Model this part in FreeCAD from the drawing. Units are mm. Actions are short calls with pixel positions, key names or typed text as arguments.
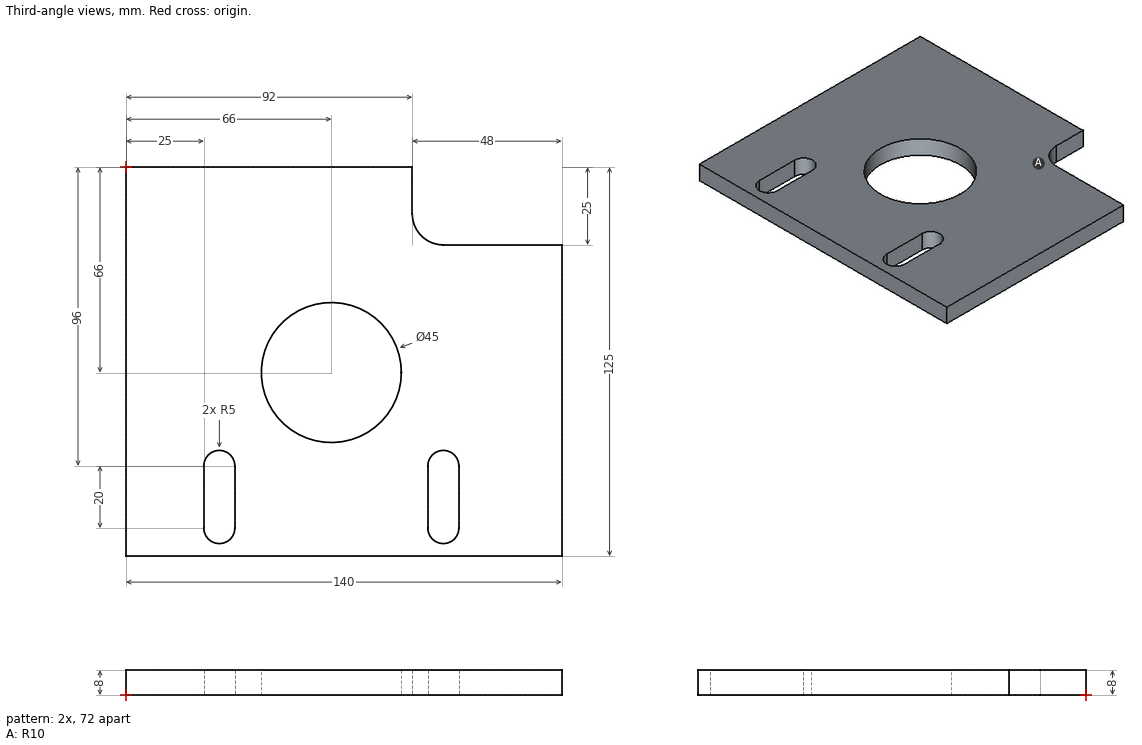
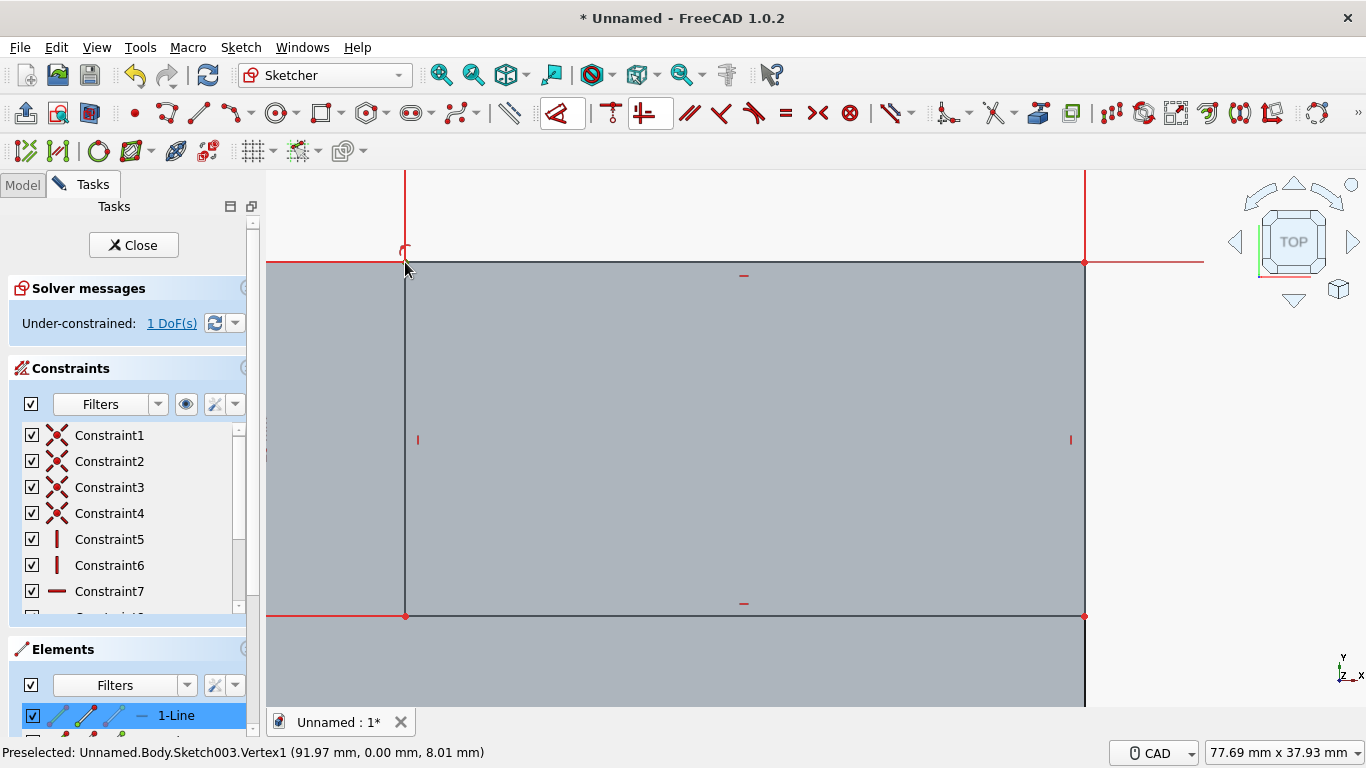
key(l)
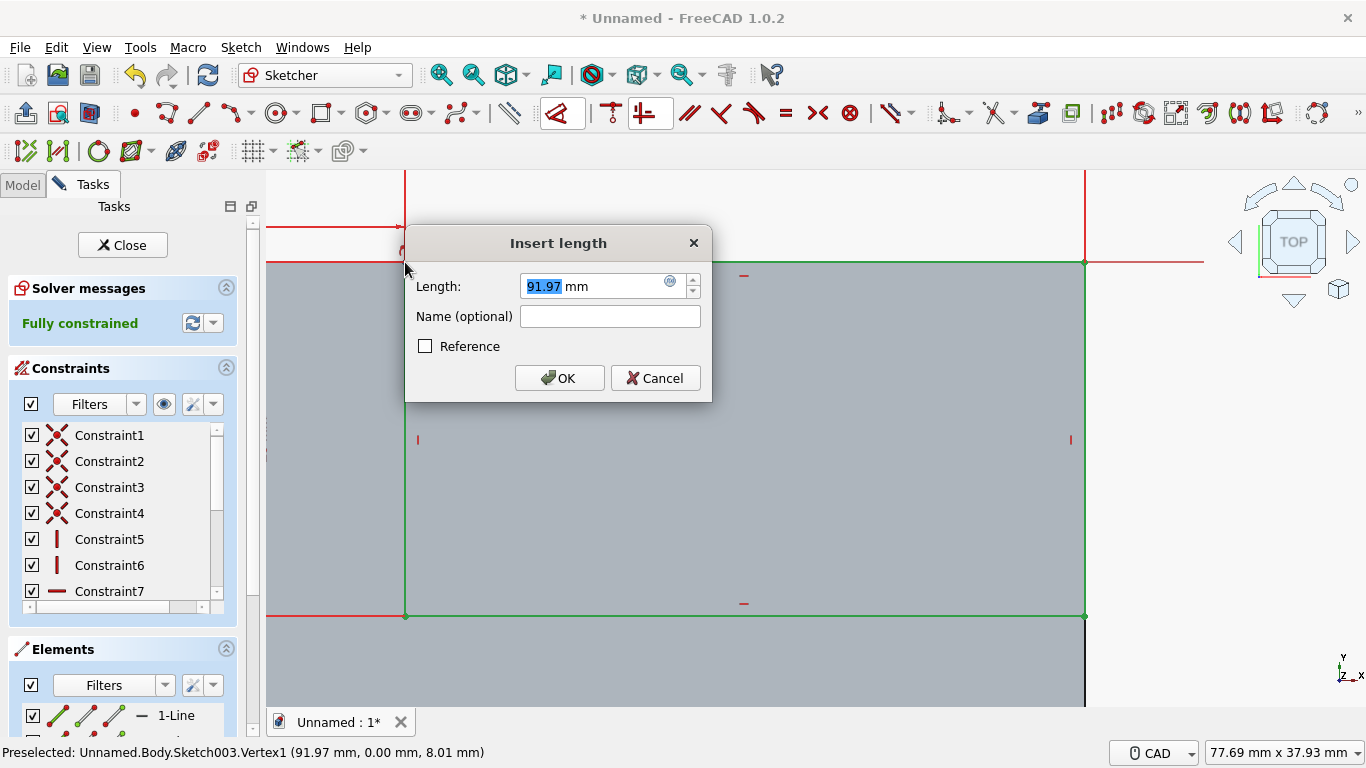
text(92)
key(Return)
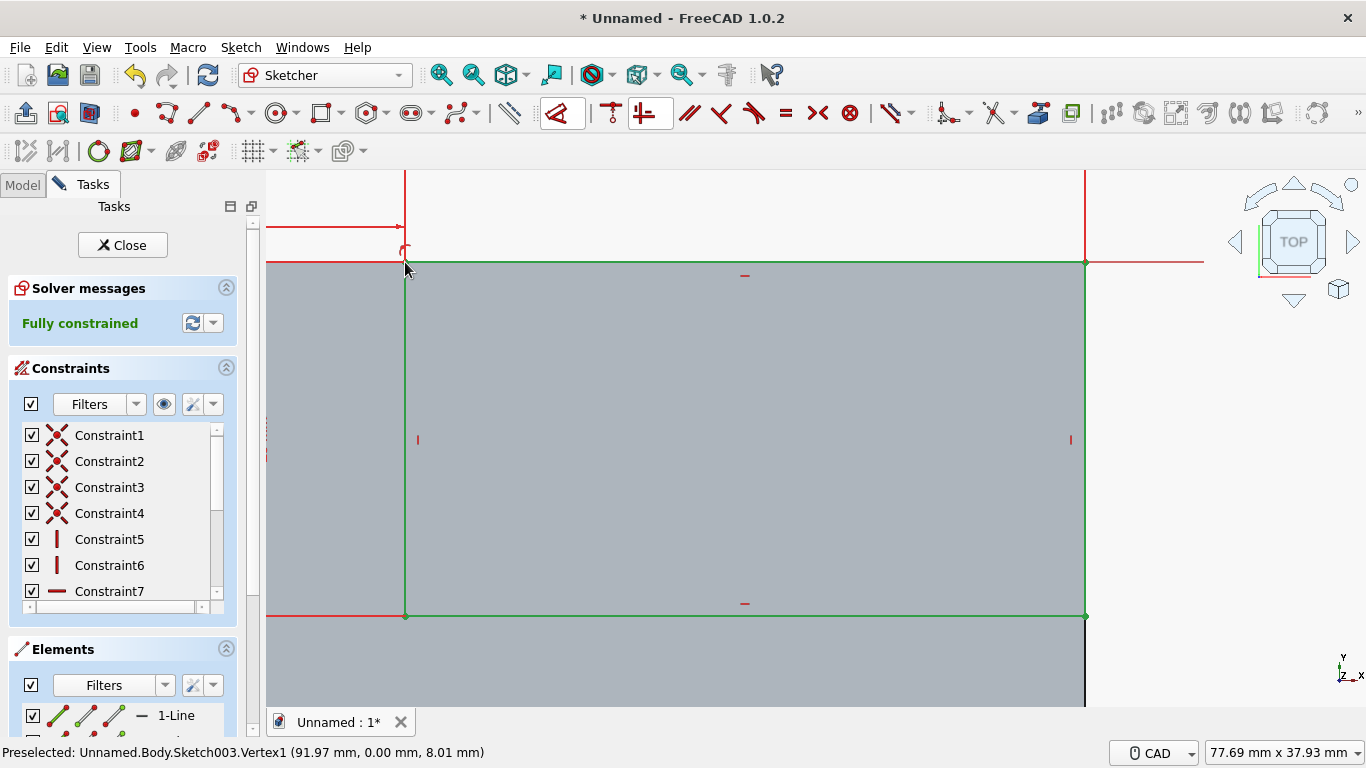
click(123, 245)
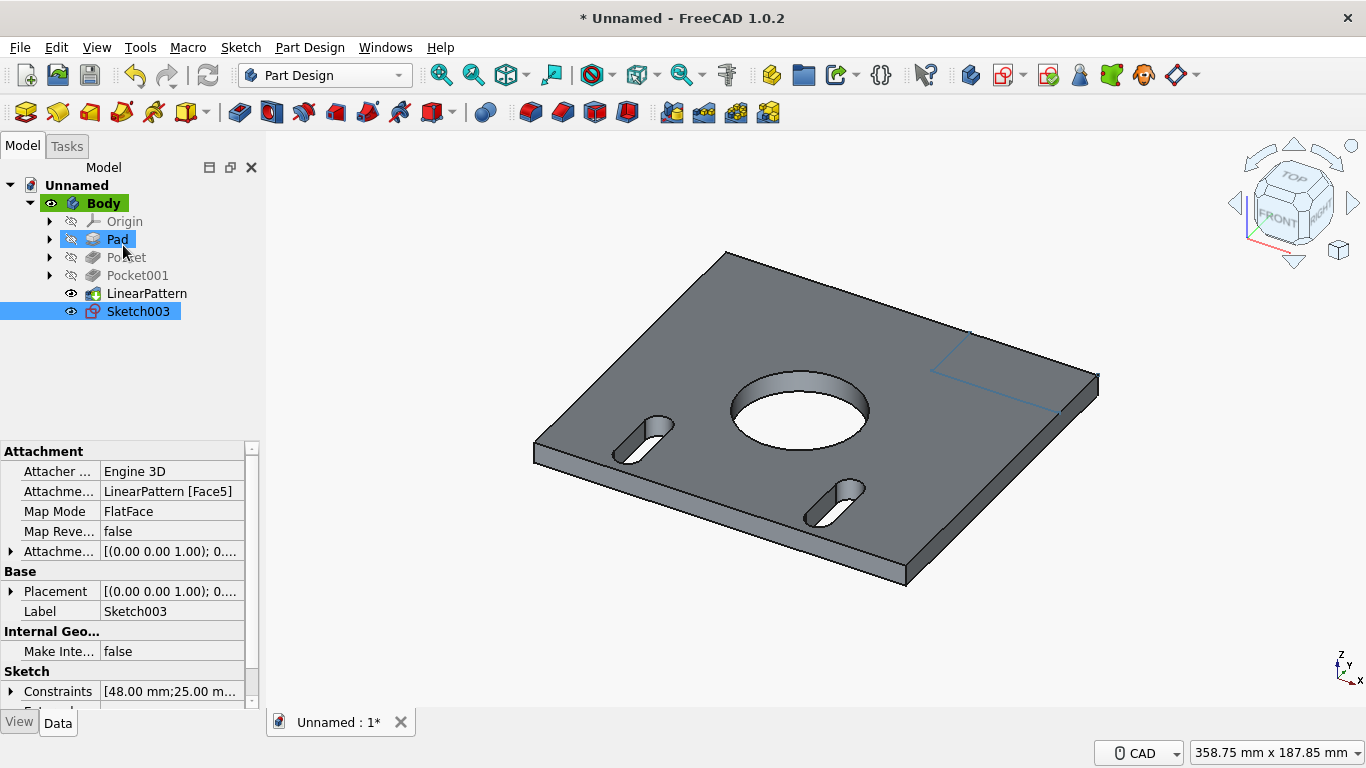
click(240, 112)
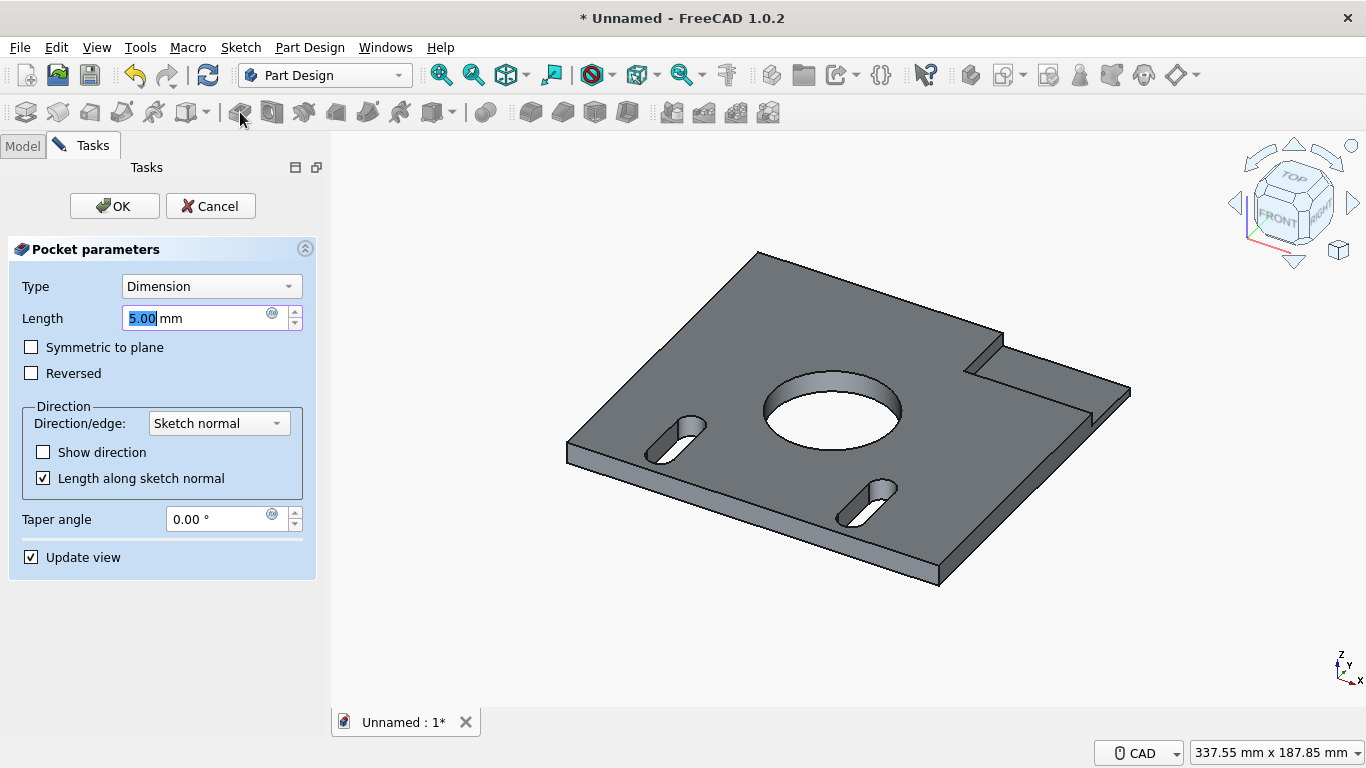
text(8)
key(Tab)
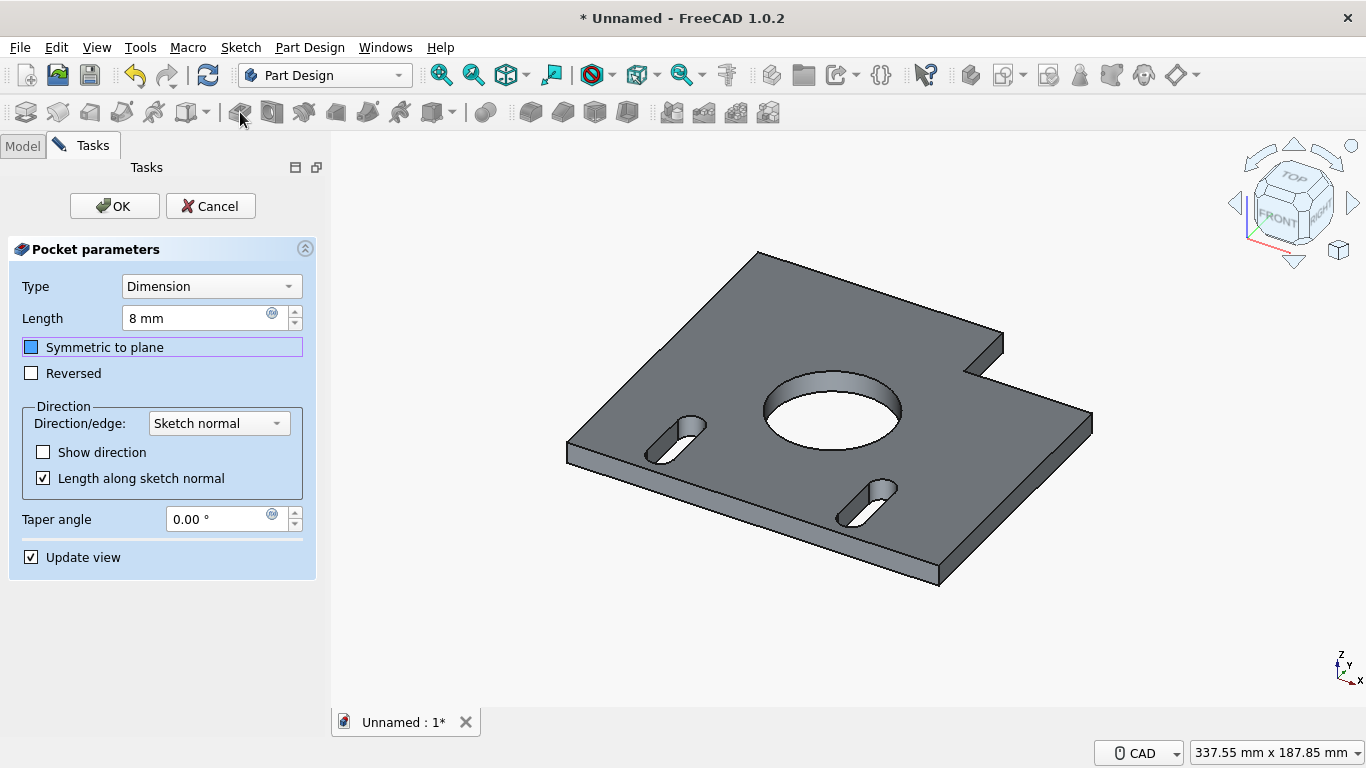
click(115, 206)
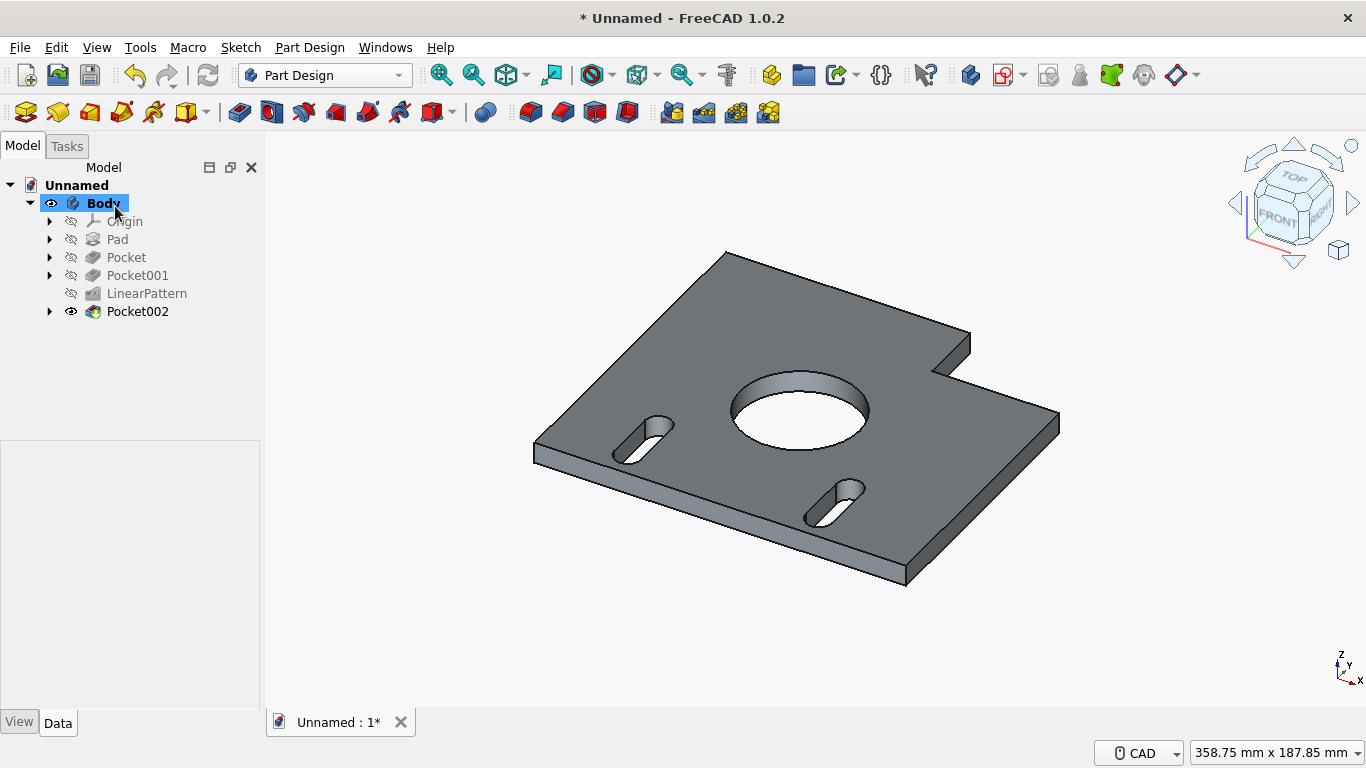
key(0)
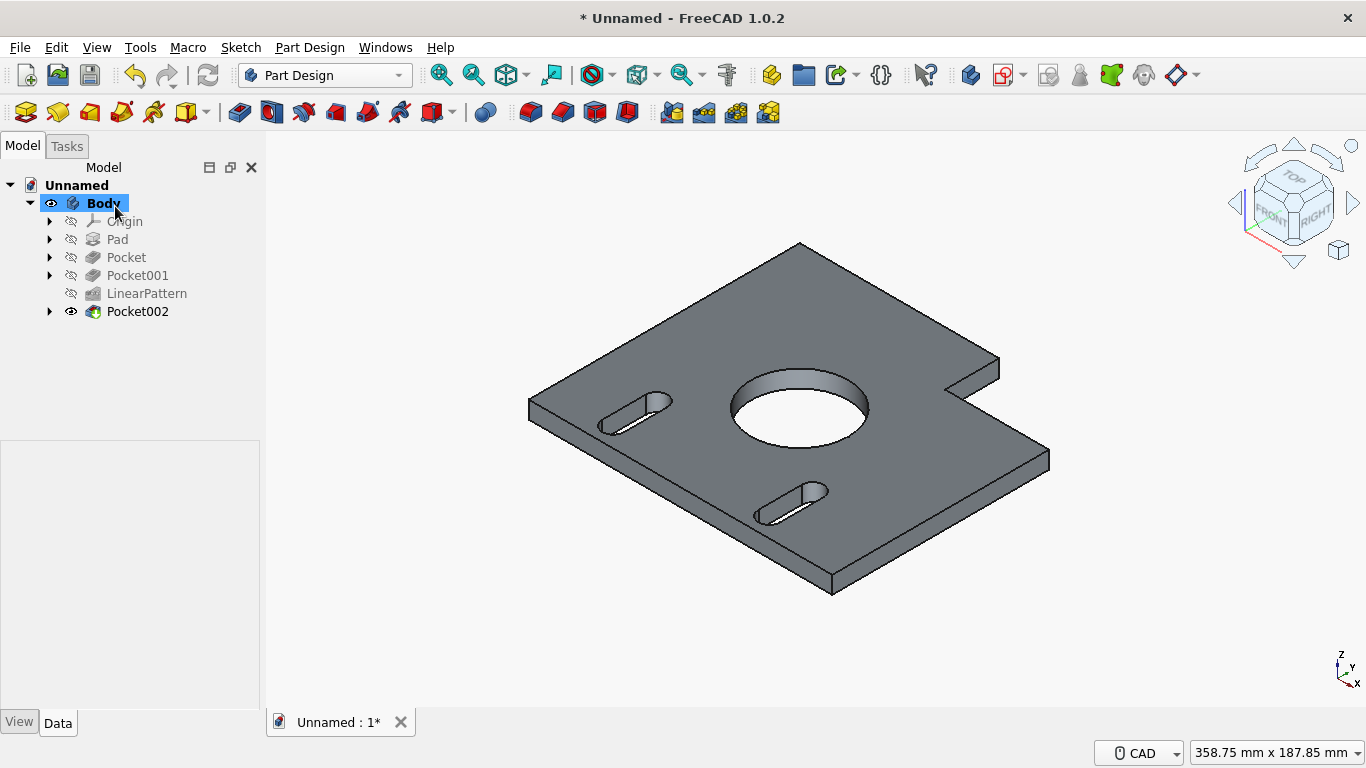
key(2)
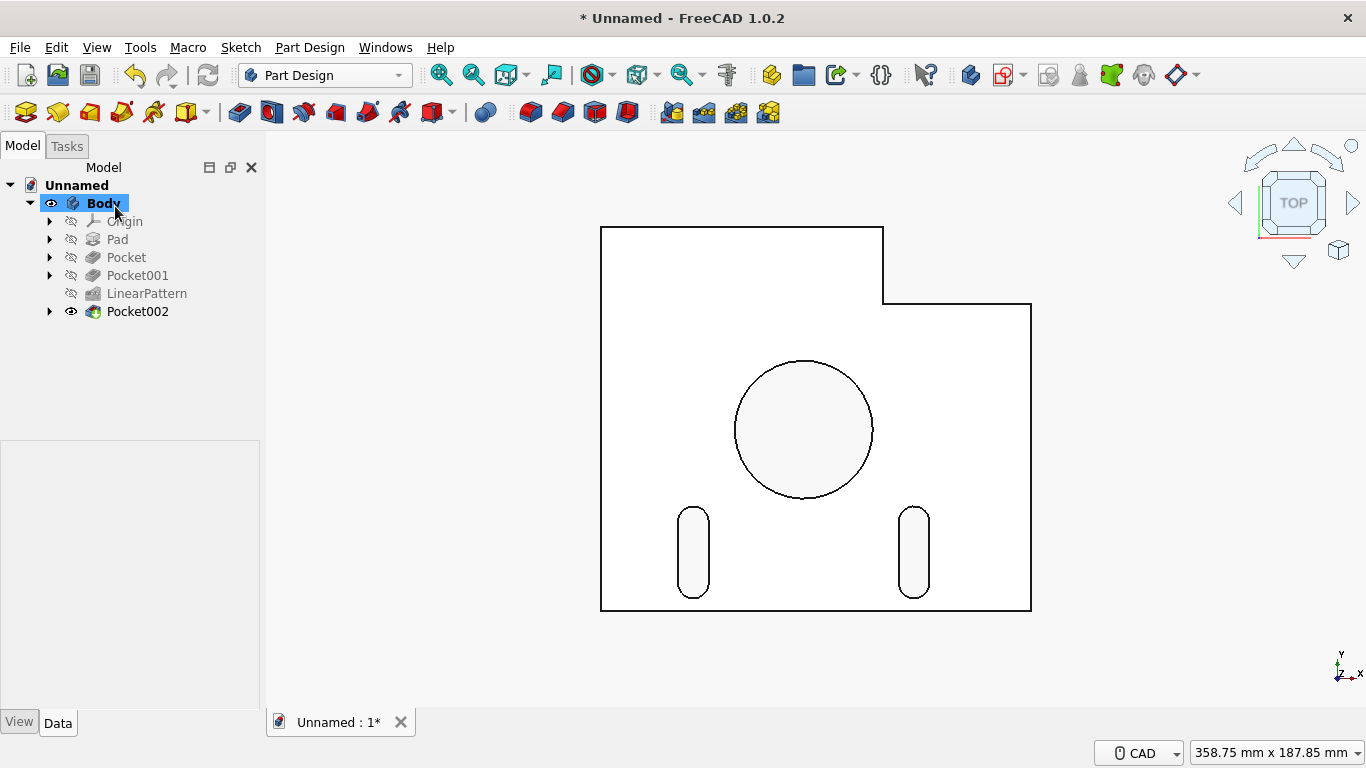
key(1)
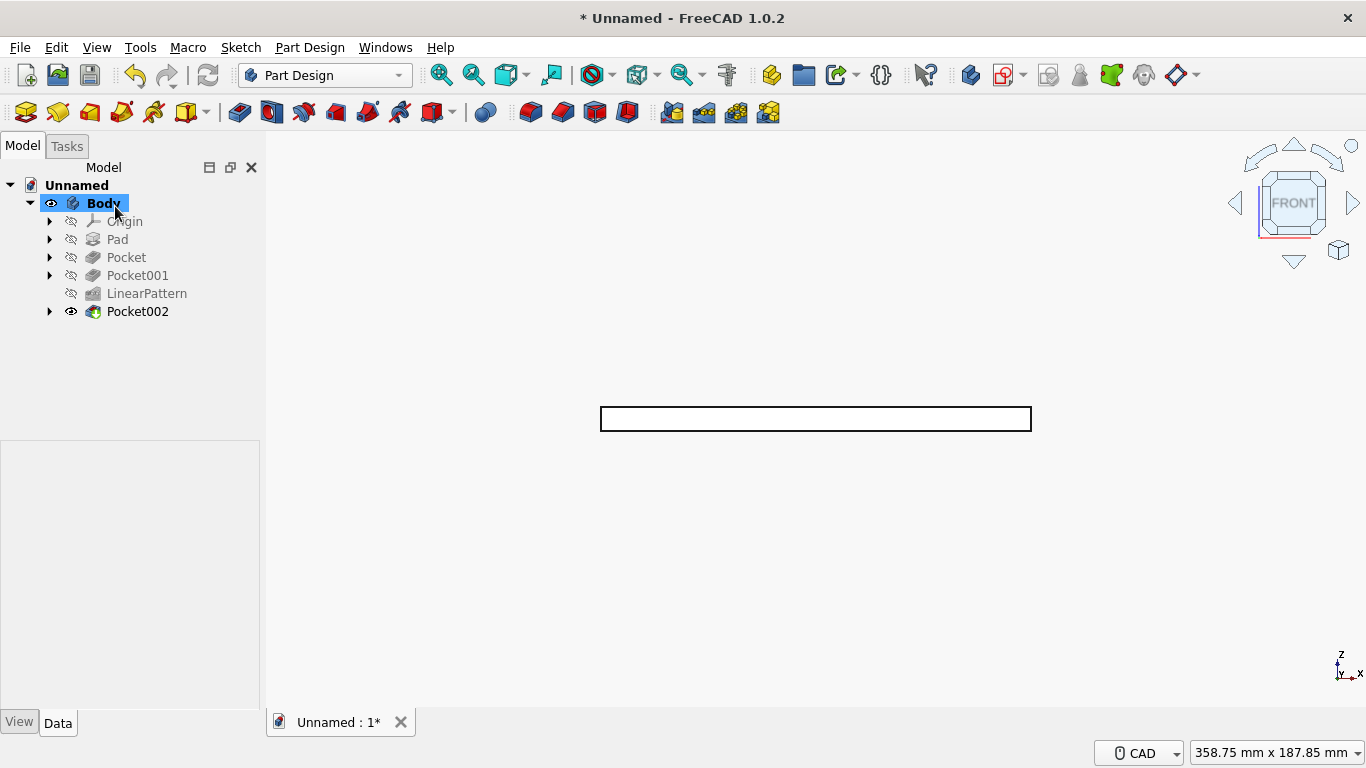
click(442, 76)